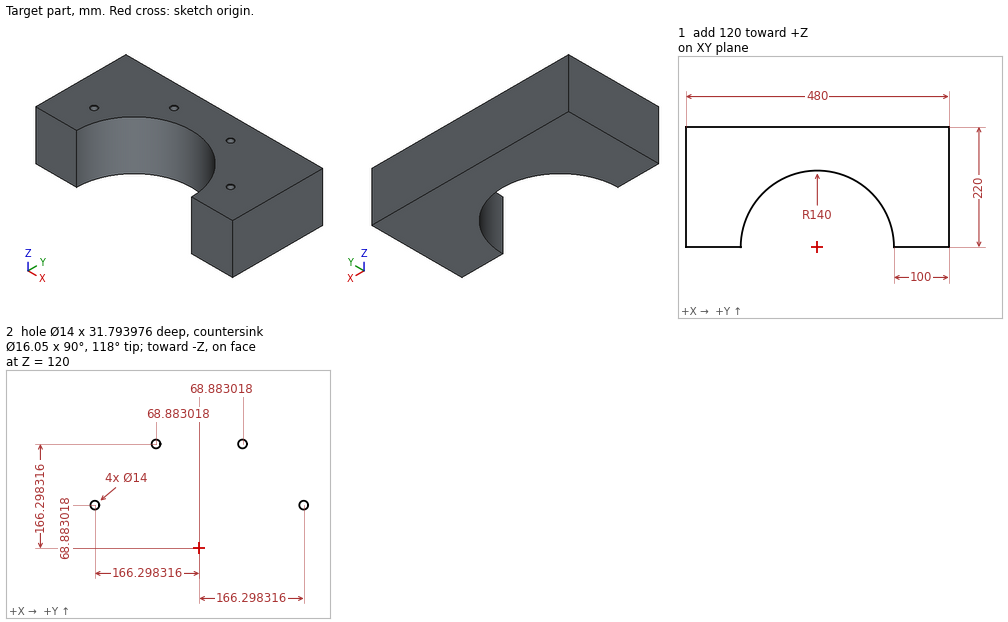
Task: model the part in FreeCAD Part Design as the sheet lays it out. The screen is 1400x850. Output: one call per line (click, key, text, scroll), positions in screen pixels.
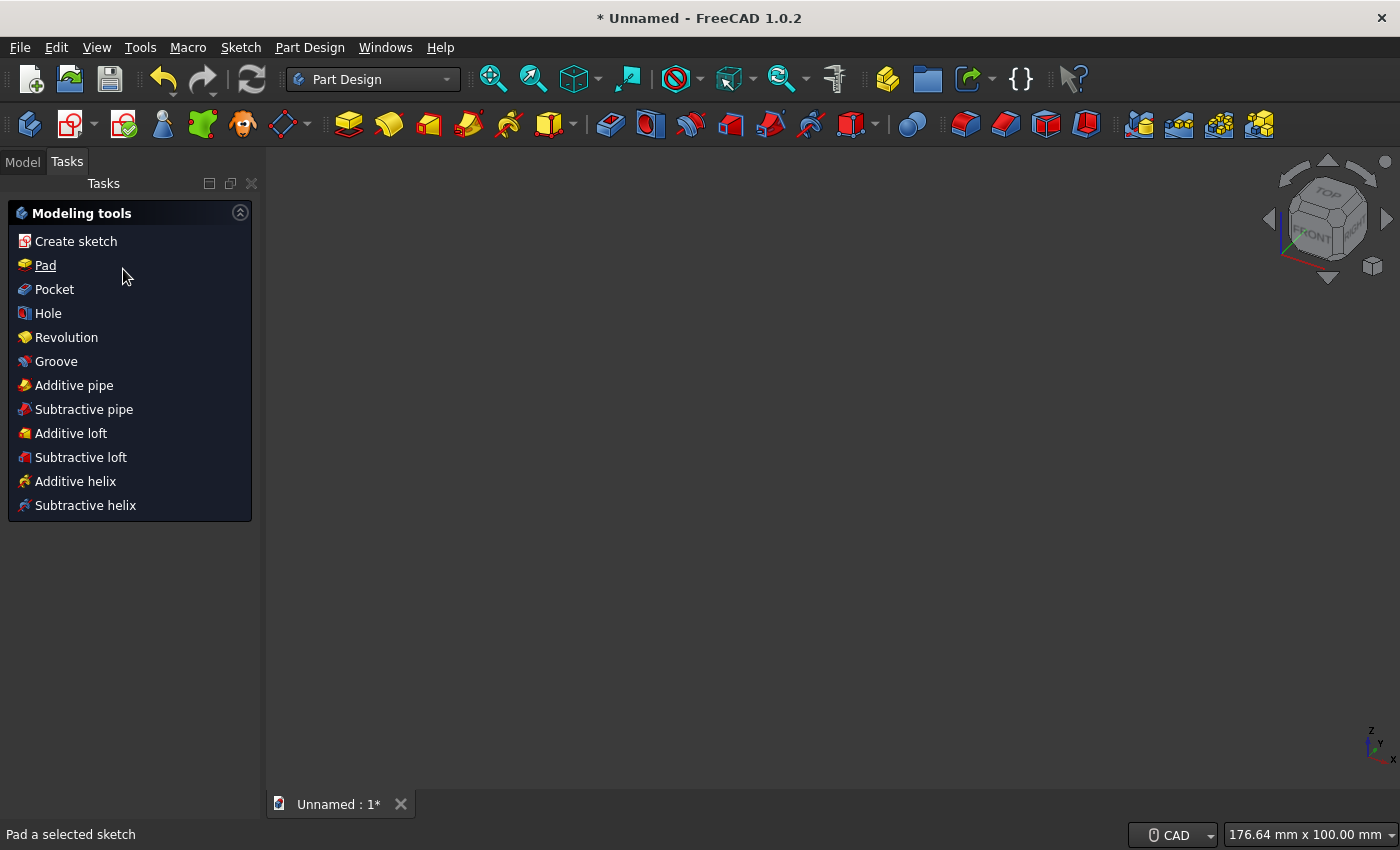
click(350, 124)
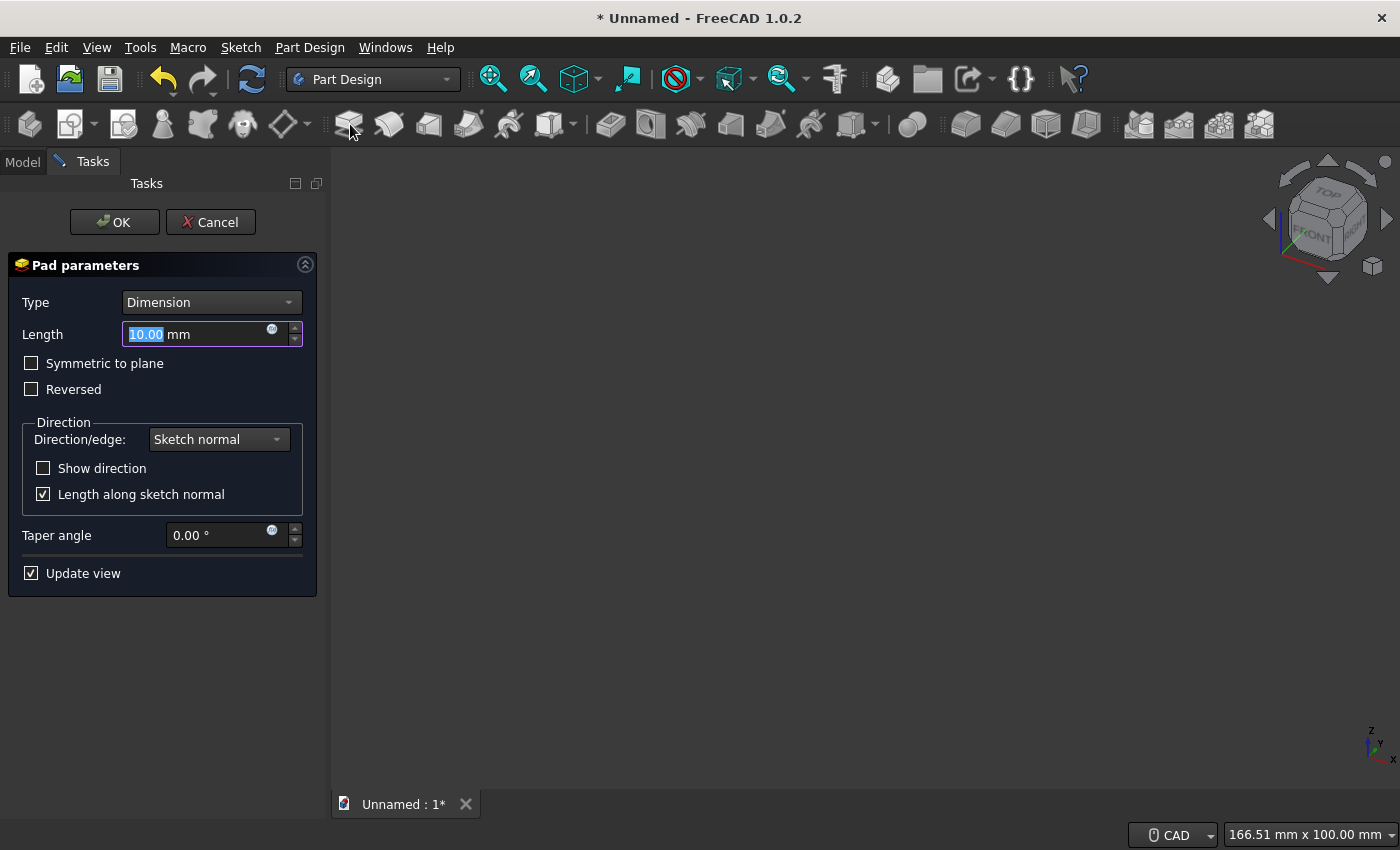
text(120)
key(Tab)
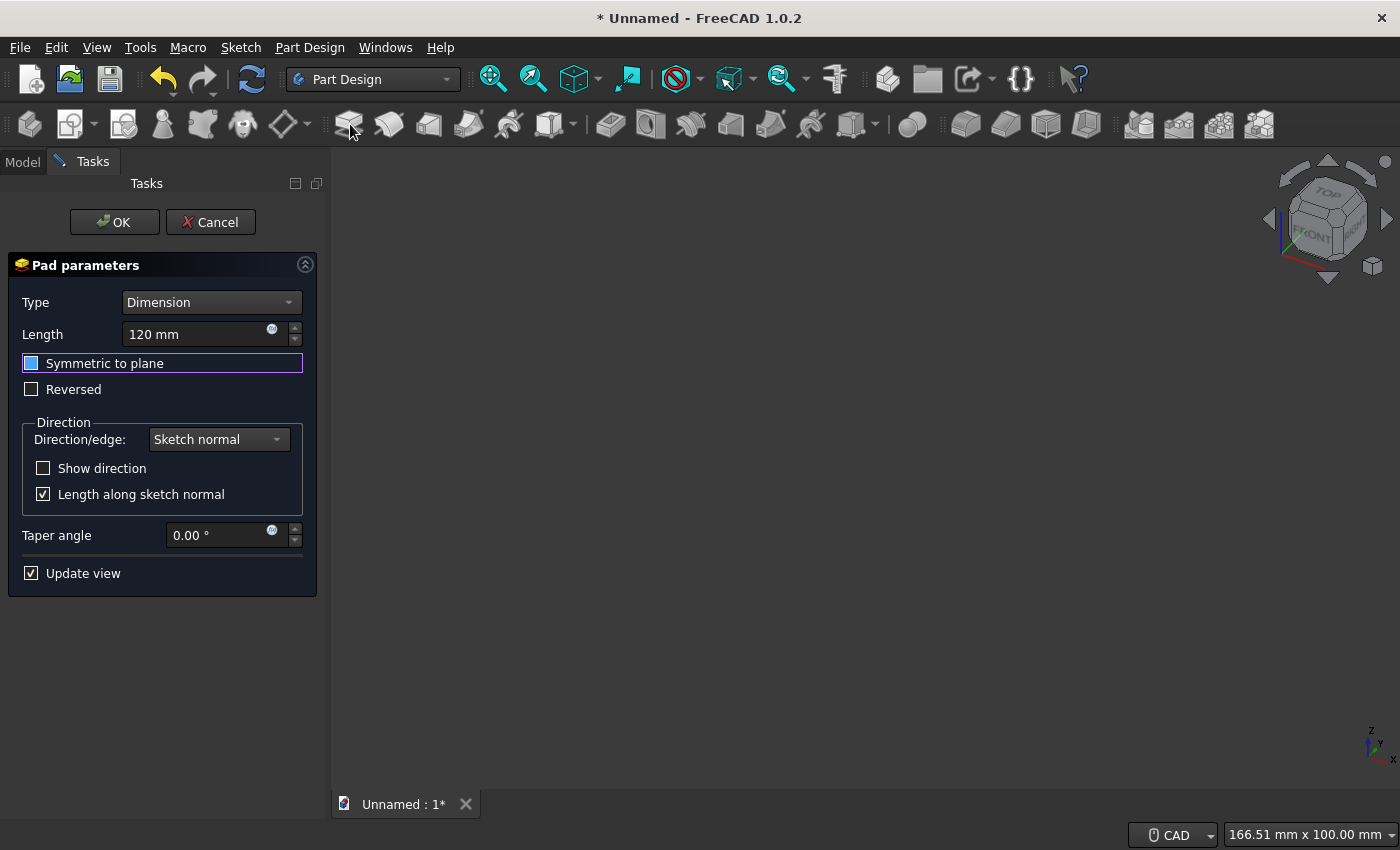
click(115, 222)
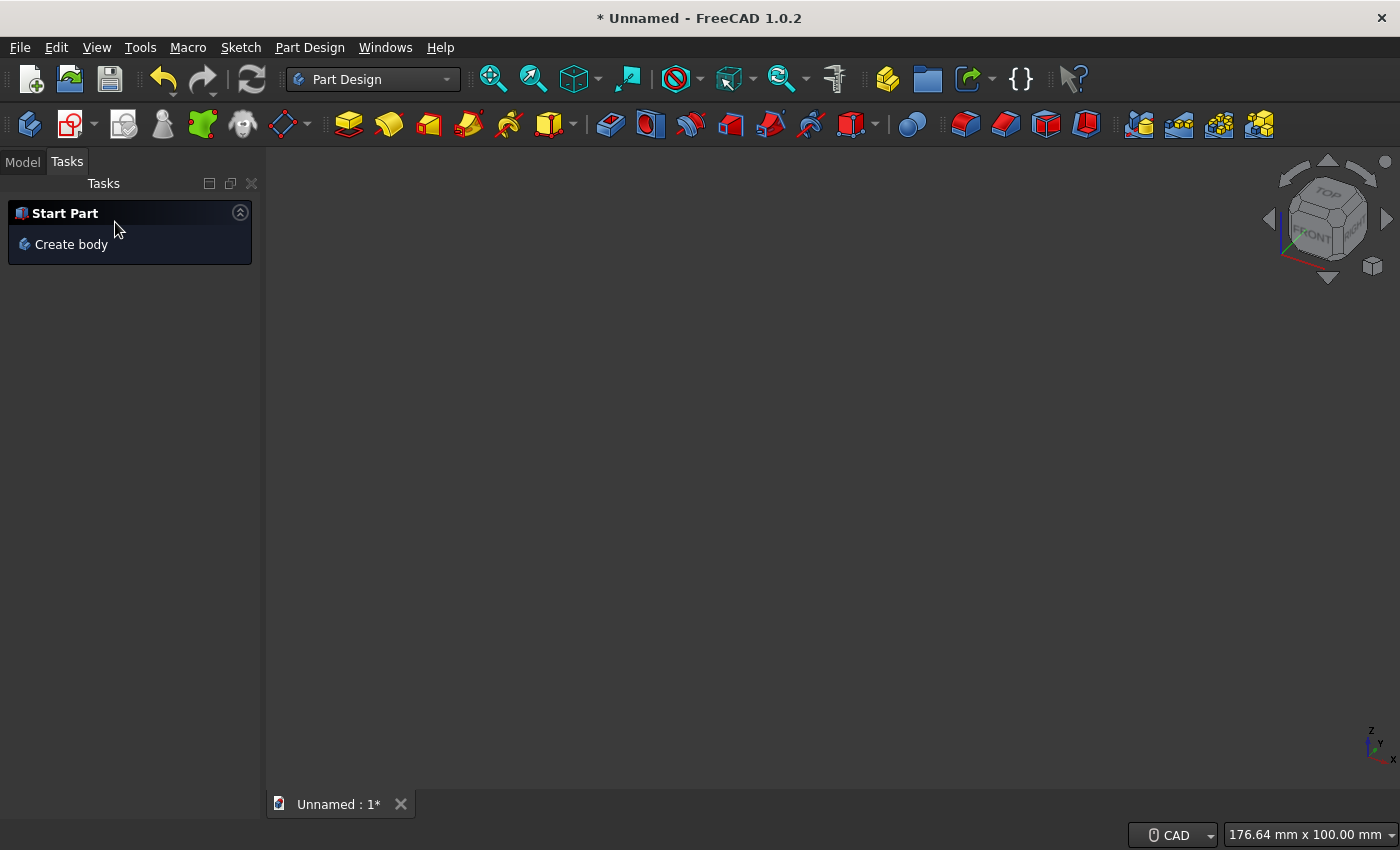
click(494, 80)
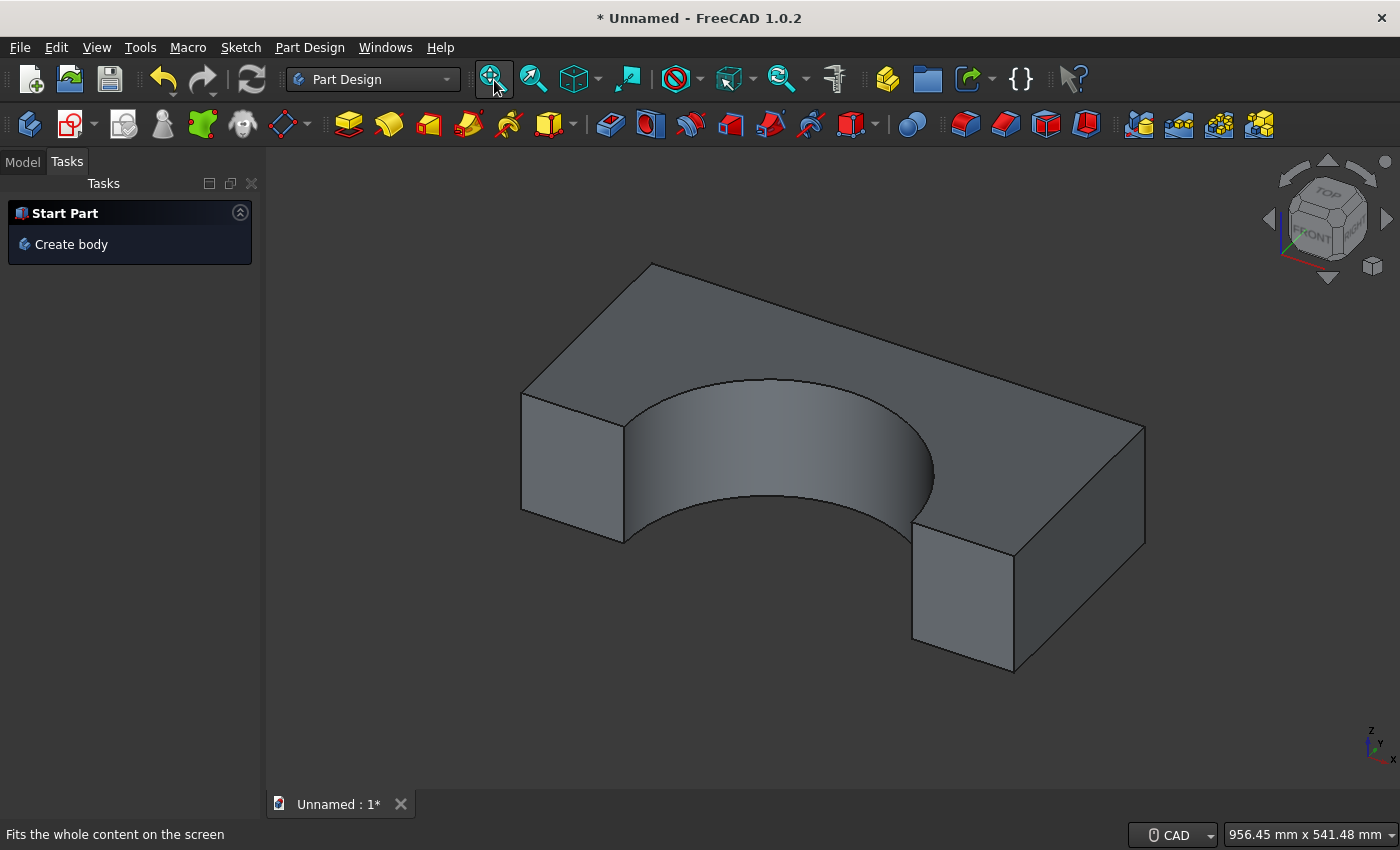
click(992, 437)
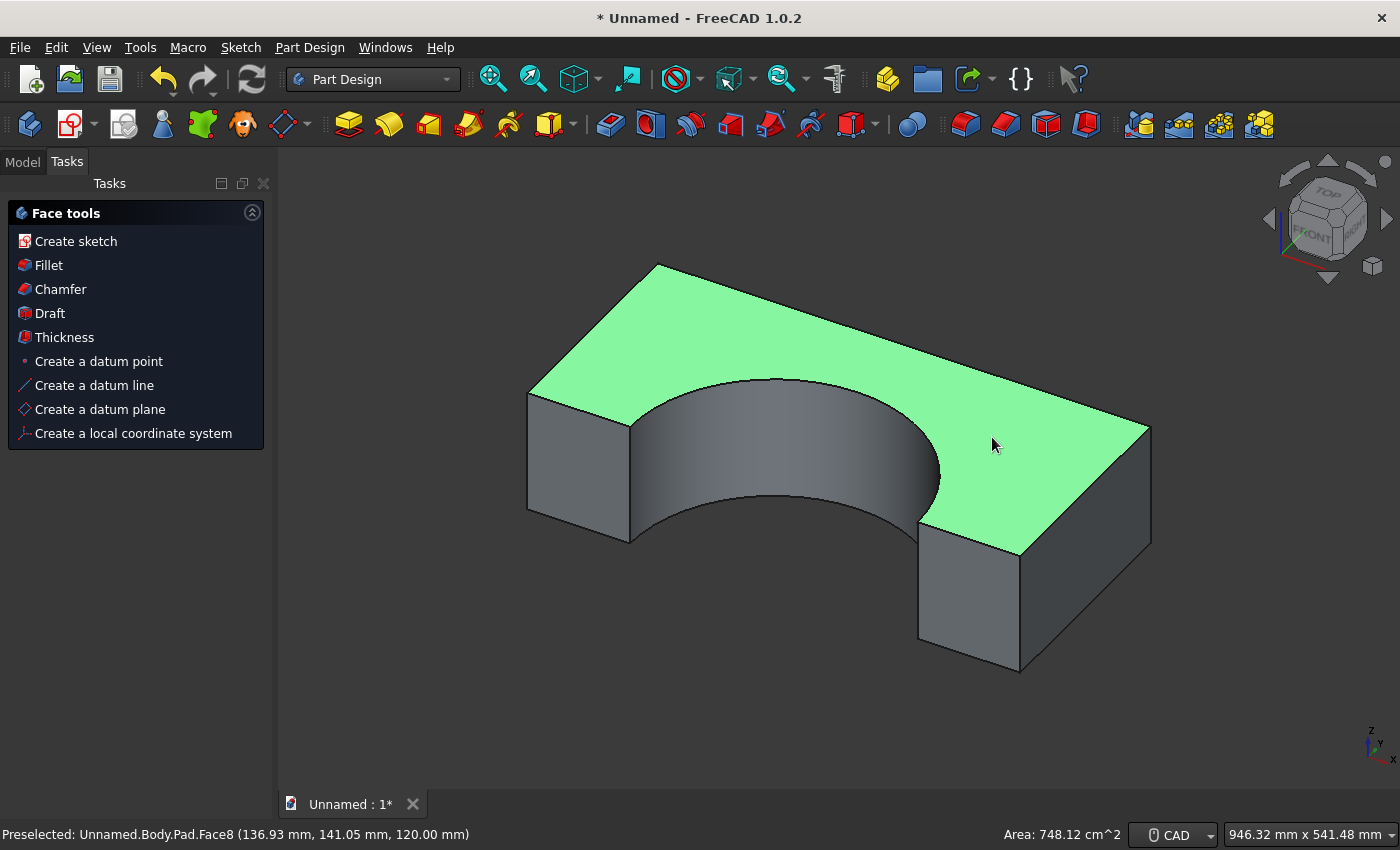
click(70, 124)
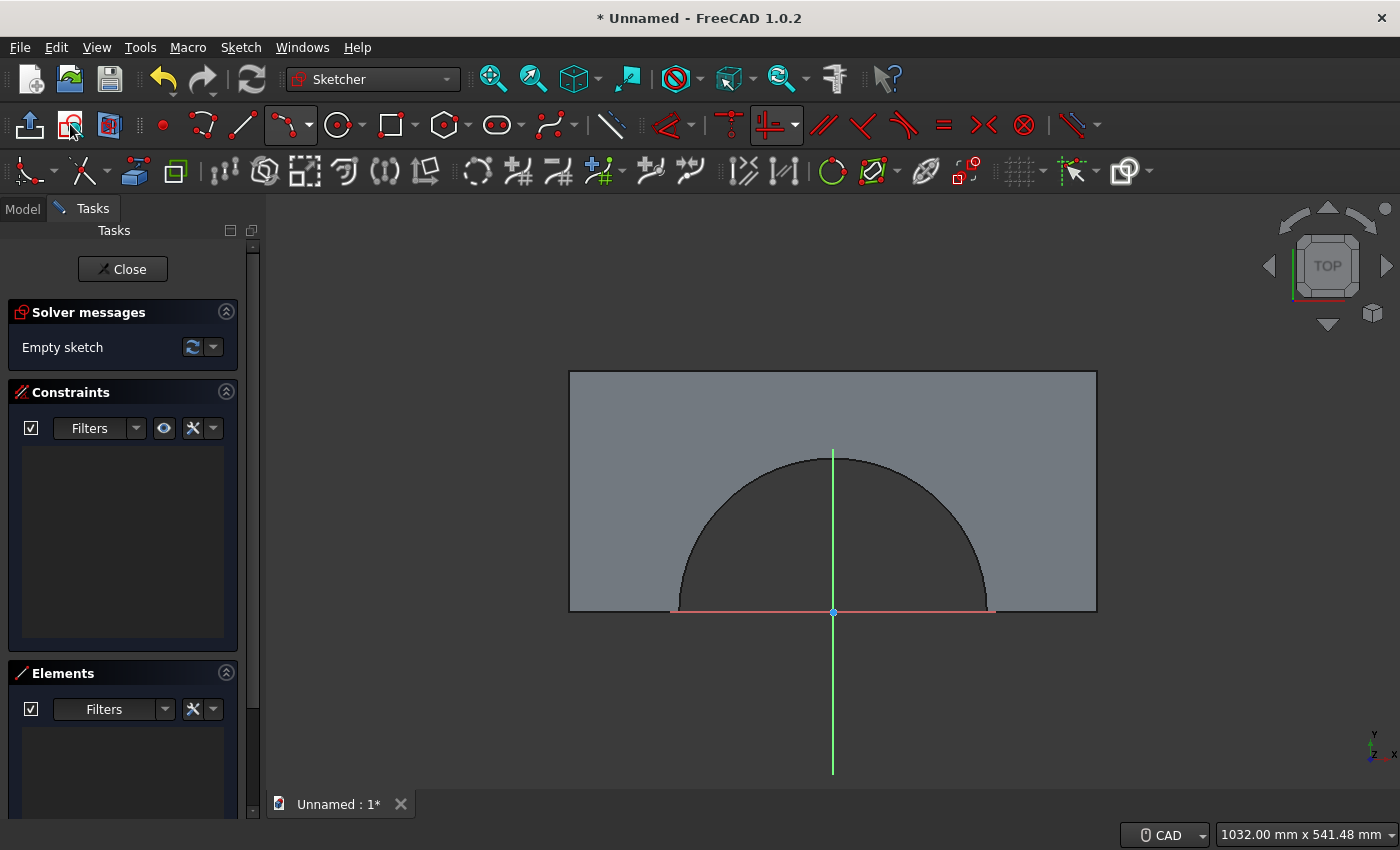
scroll(916, 548, up, 3)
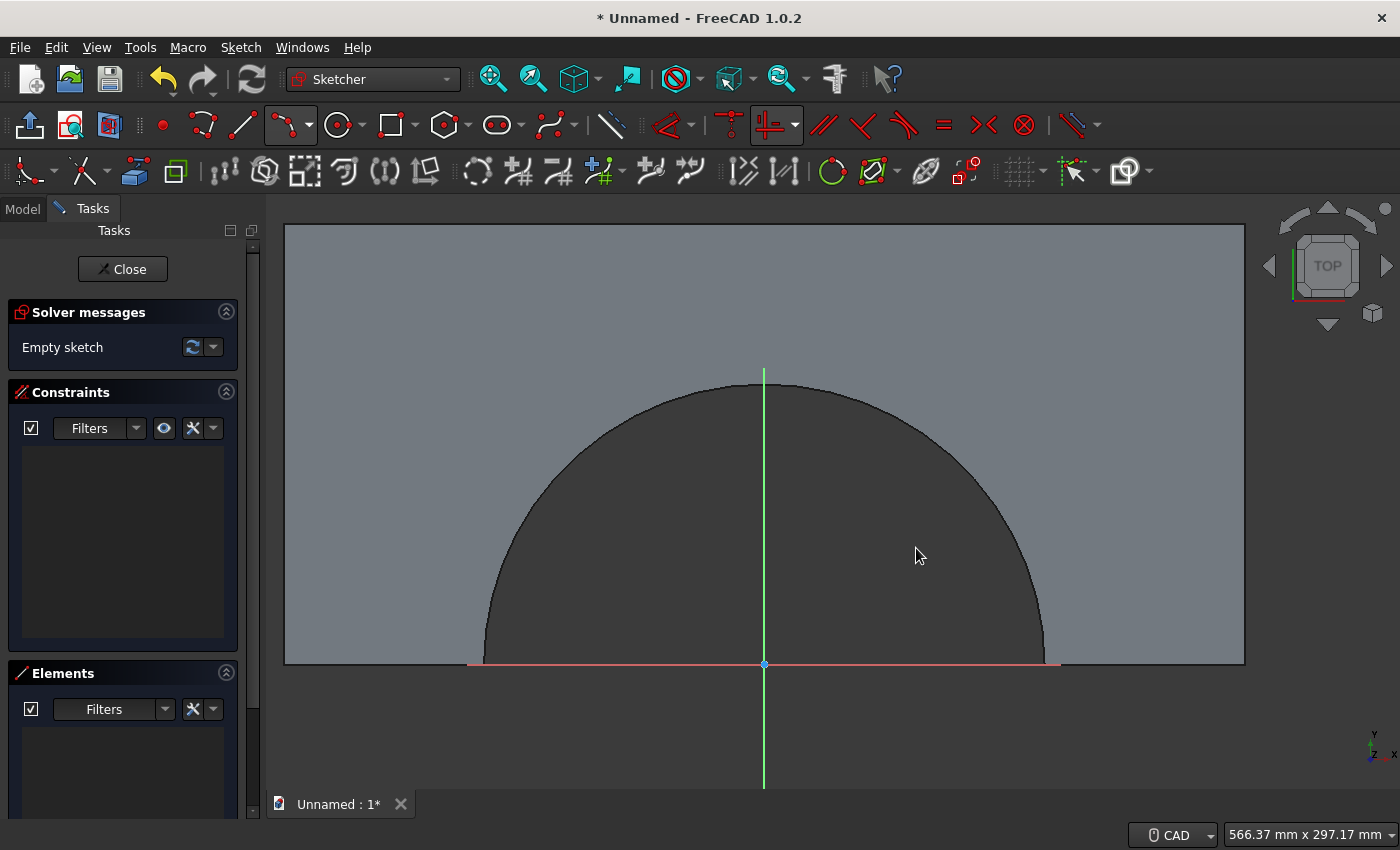
click(338, 126)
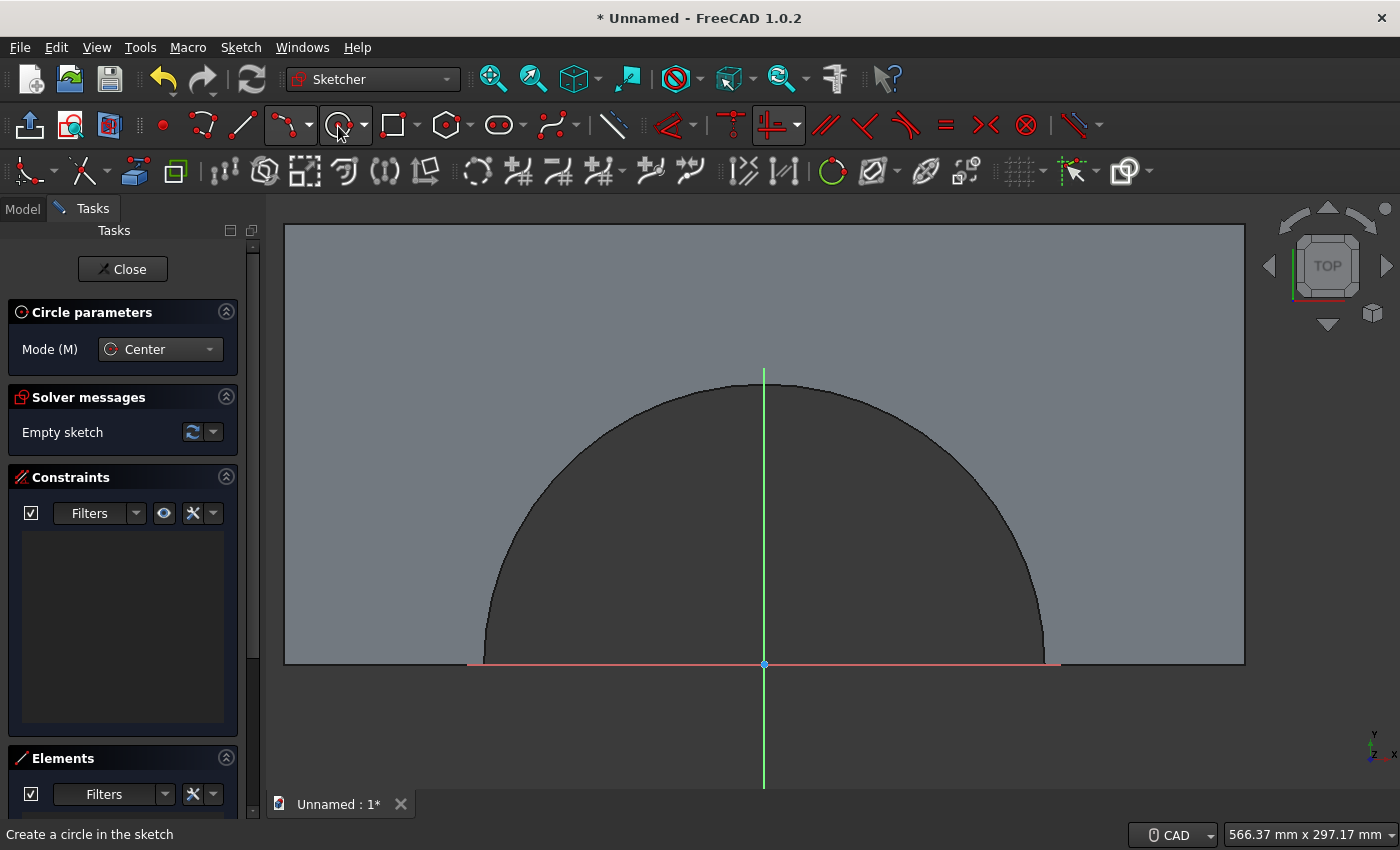
scroll(431, 527, up, 3)